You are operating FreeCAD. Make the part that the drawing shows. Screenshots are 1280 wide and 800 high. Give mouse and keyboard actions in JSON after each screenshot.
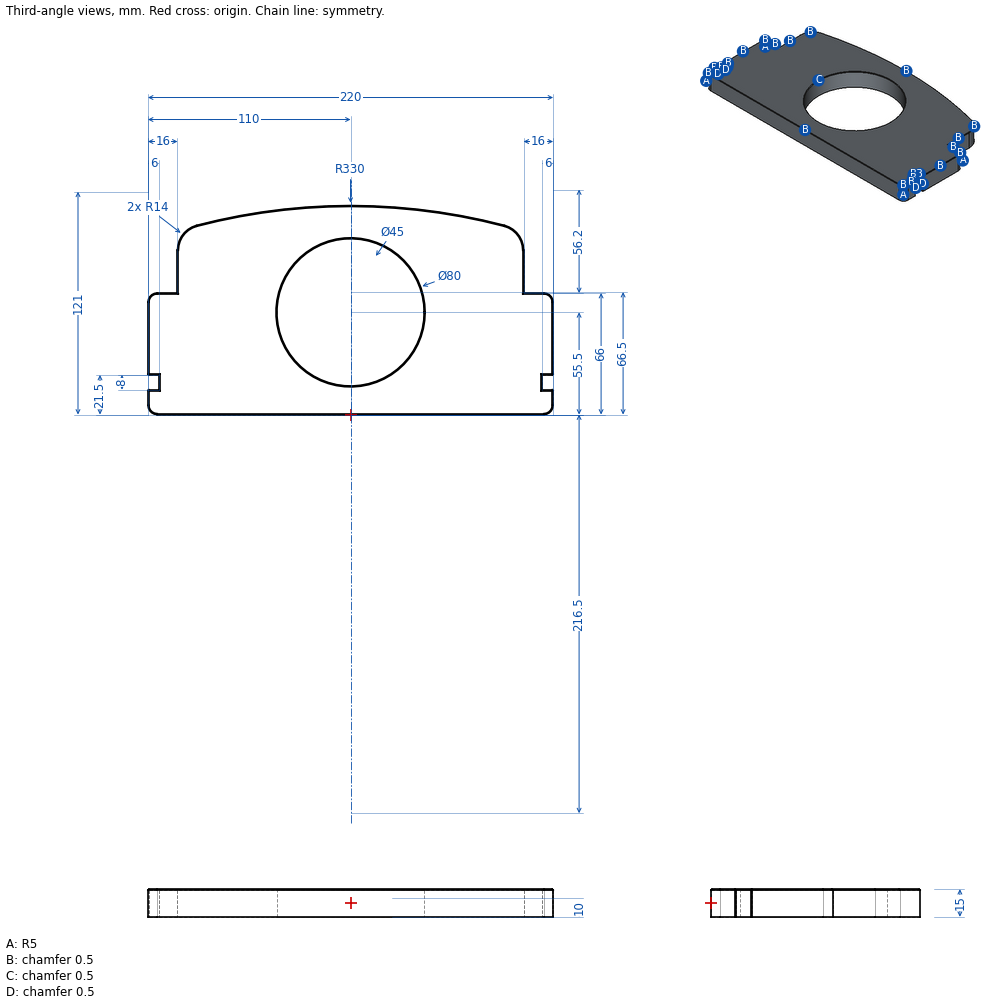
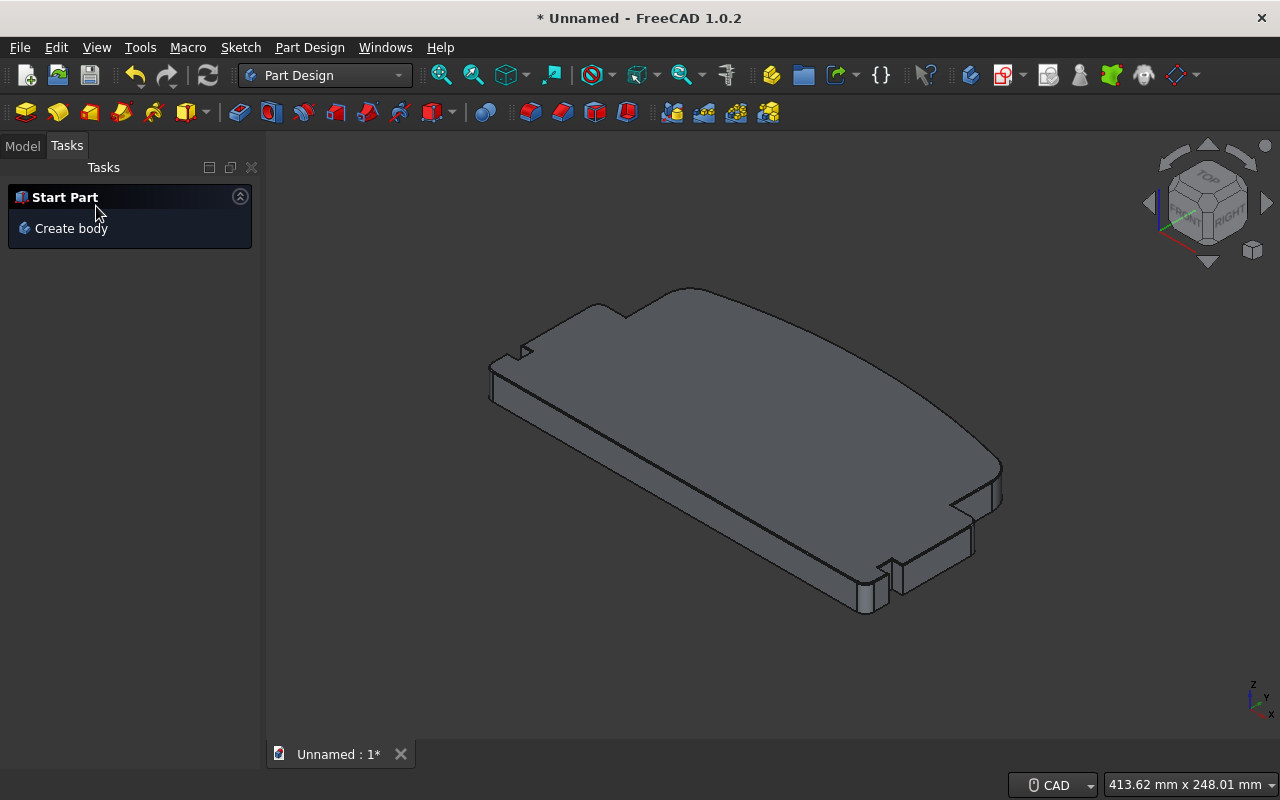
{"action": "left_click", "coordinate": [773, 419]}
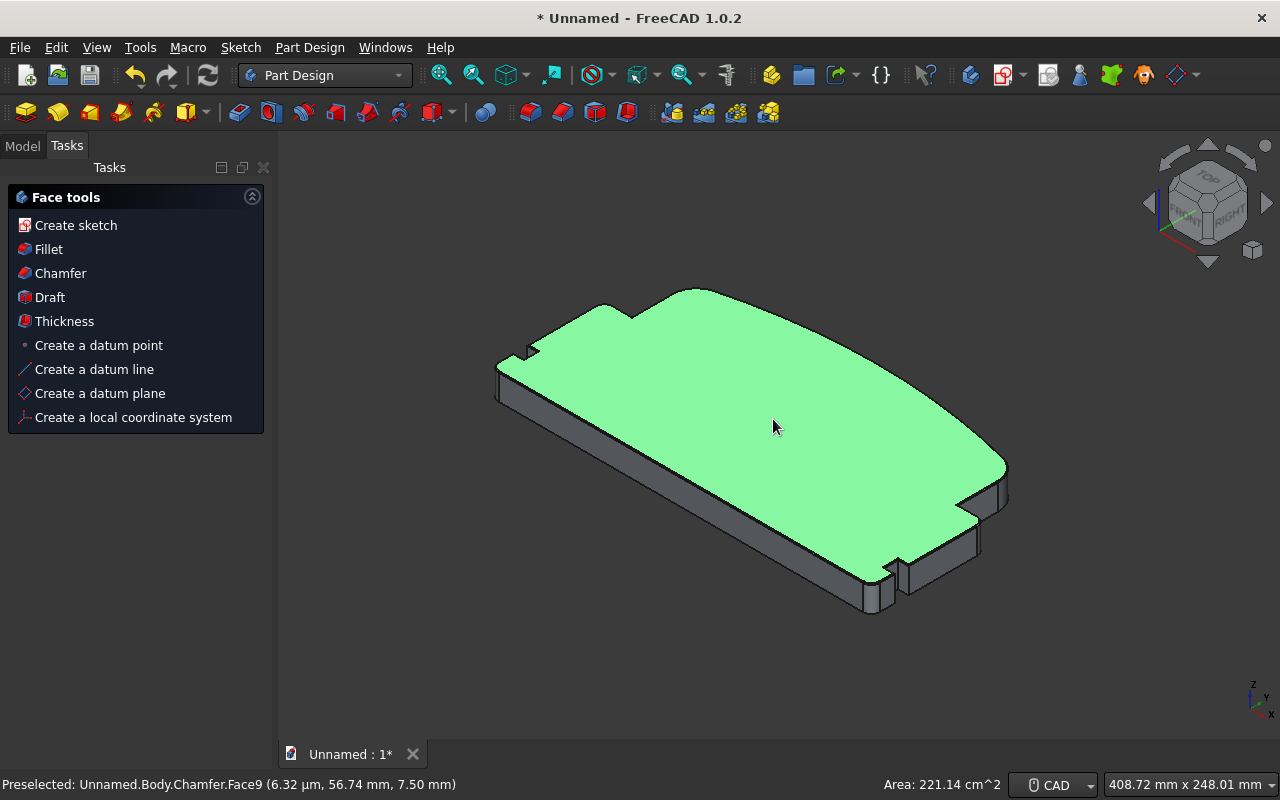
{"action": "left_click", "coordinate": [1004, 76]}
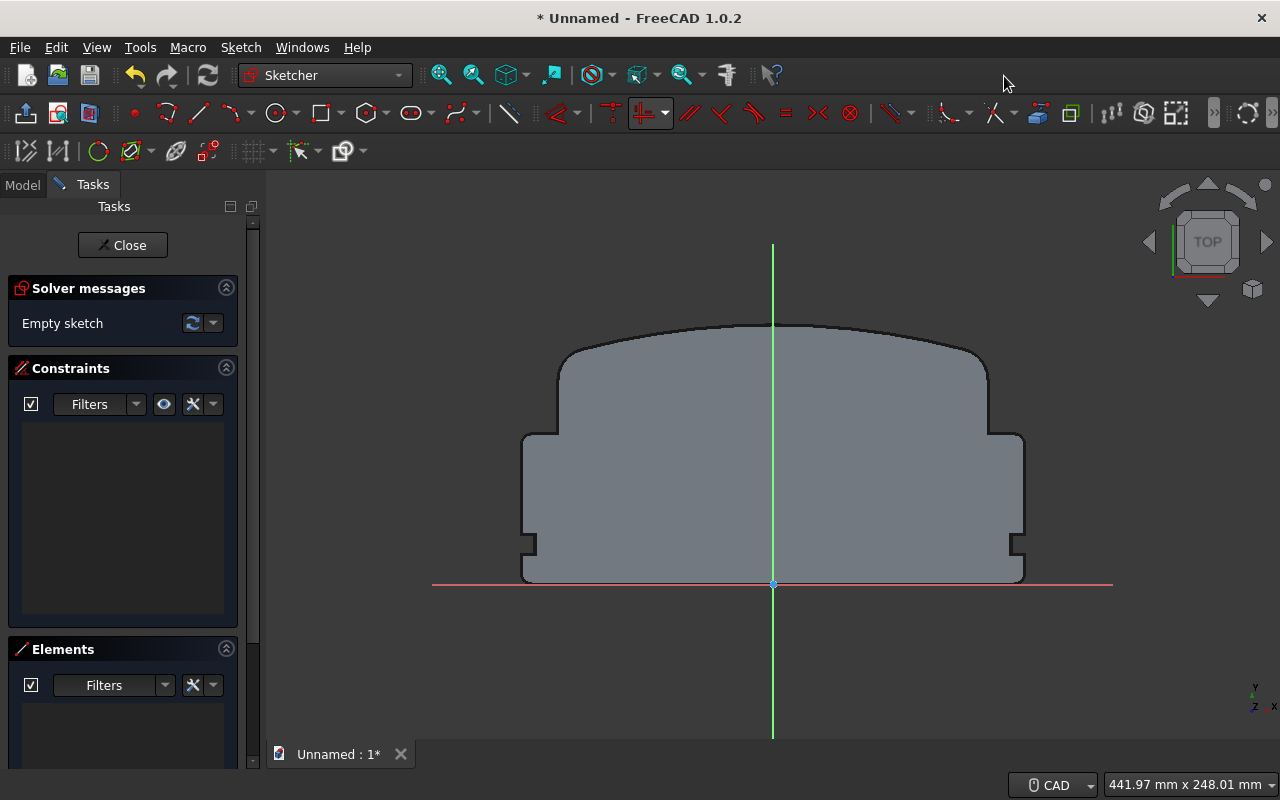
{"action": "scroll", "coordinate": [856, 500], "scroll_direction": "up", "scroll_amount": 3}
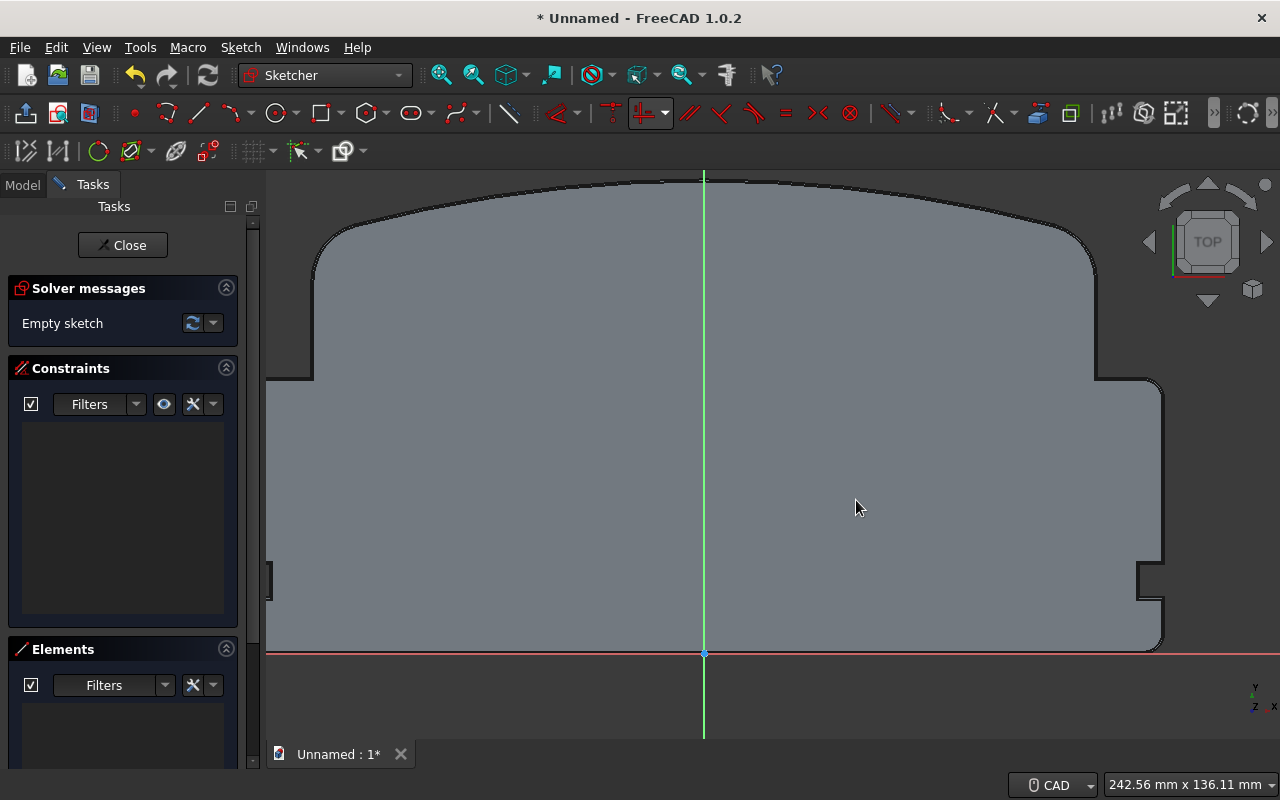
{"action": "left_click", "coordinate": [276, 114]}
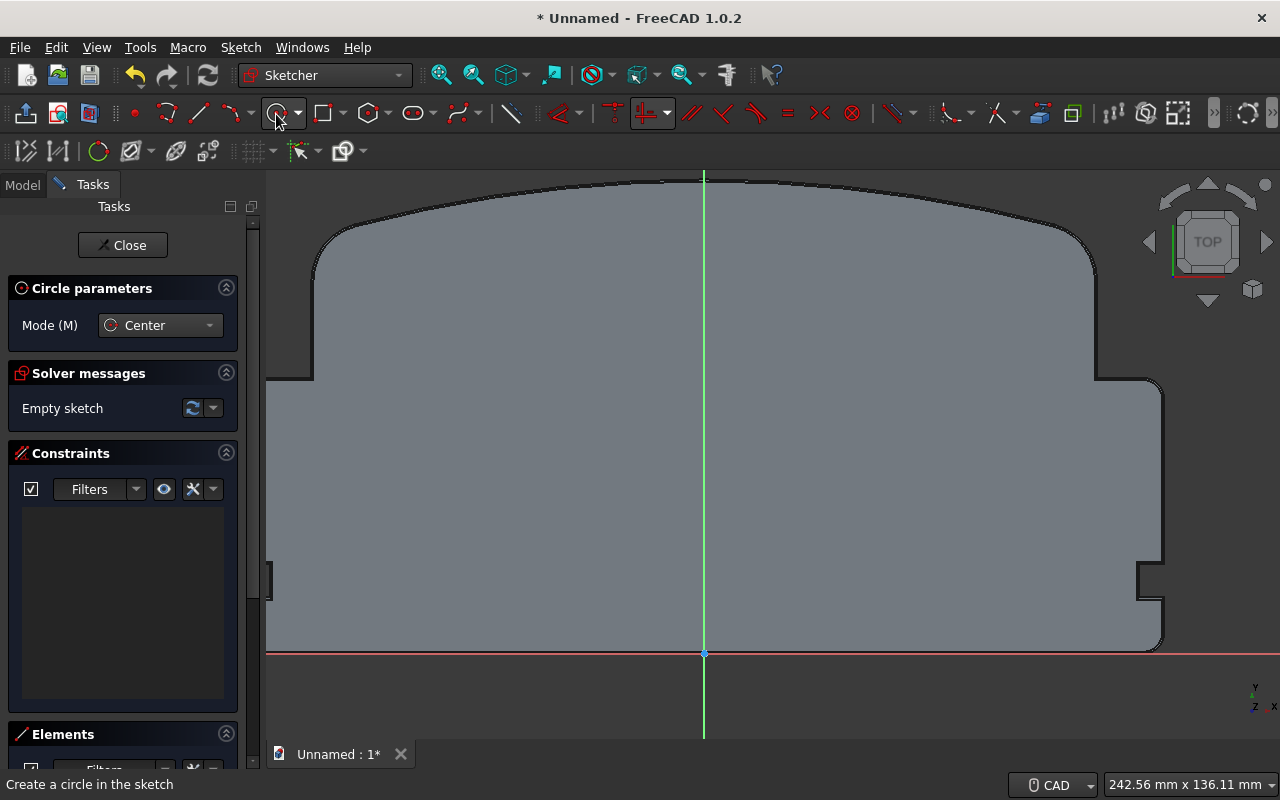
{"action": "left_click", "coordinate": [704, 422]}
{"action": "mouse_move", "coordinate": [823, 304]}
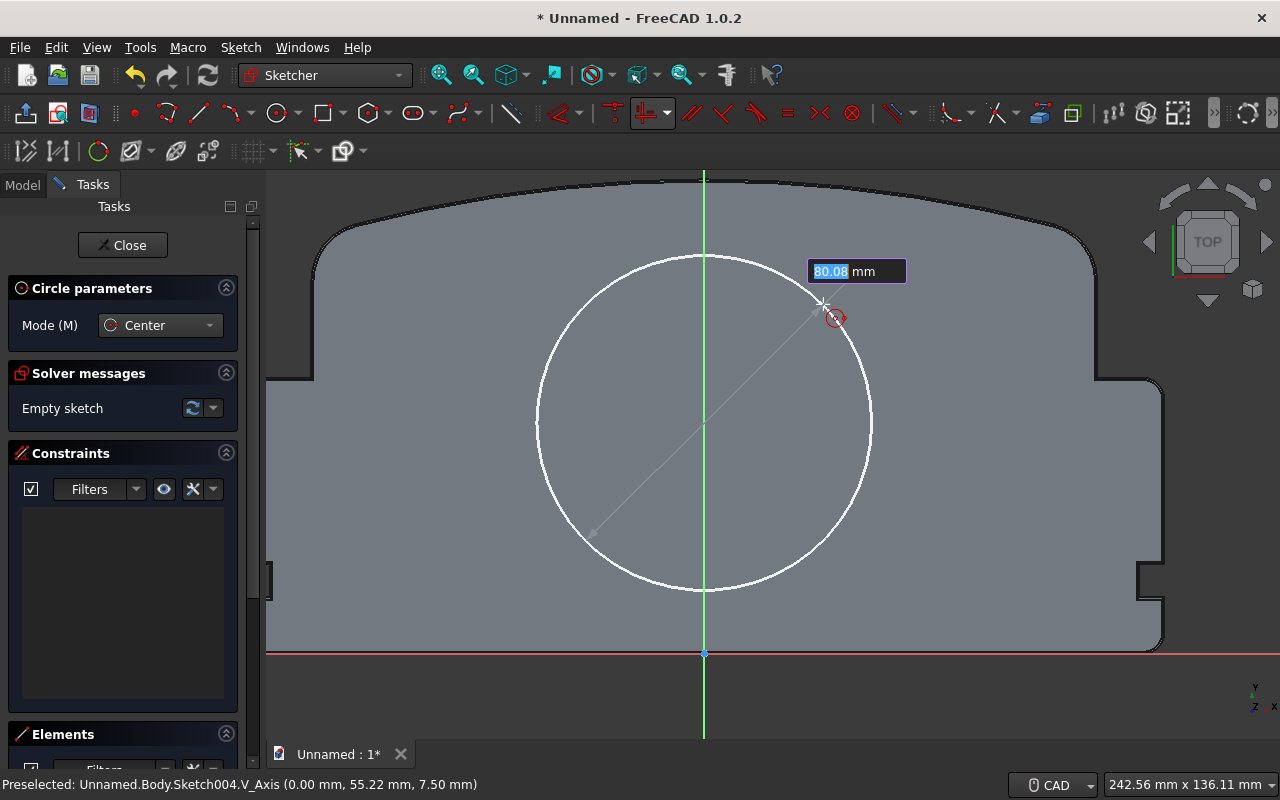
{"action": "type", "text": "80"}
{"action": "key", "text": "Return"}
{"action": "key", "text": "Escape"}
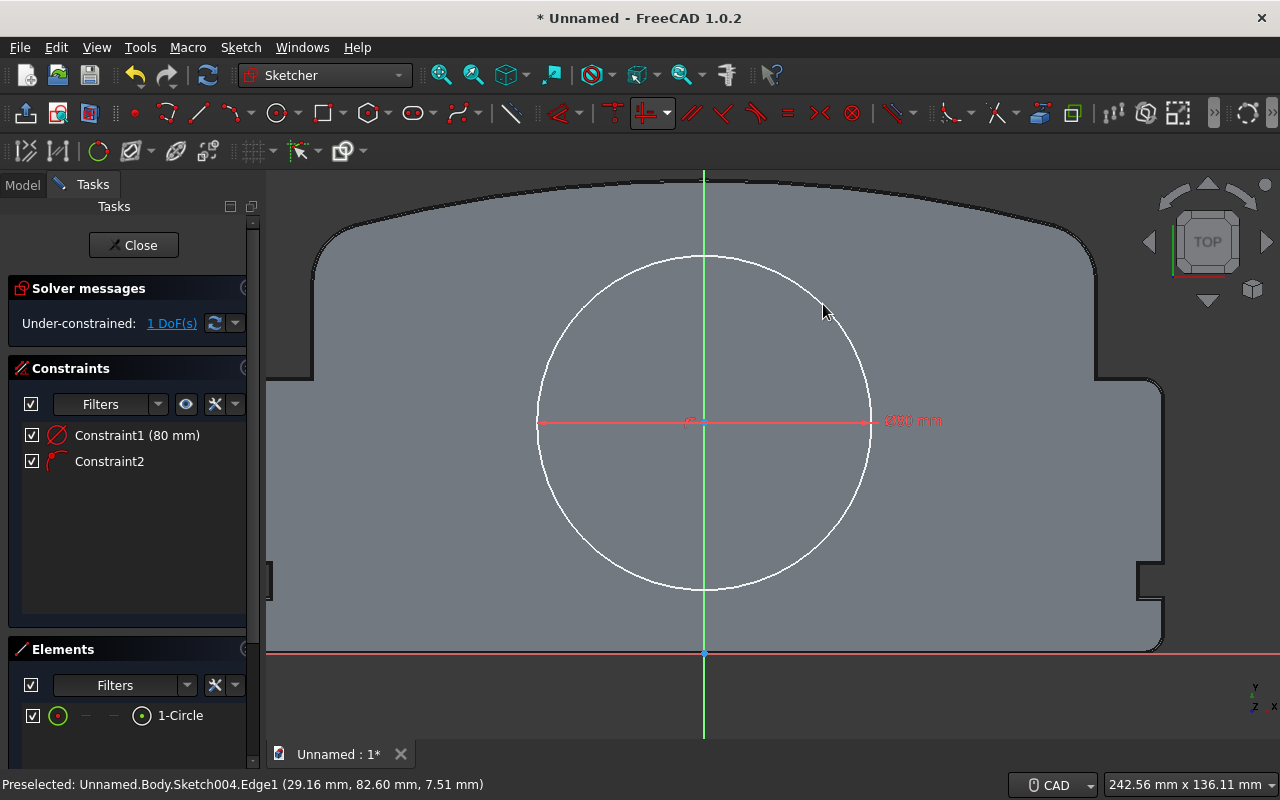
{"action": "left_click", "coordinate": [558, 114]}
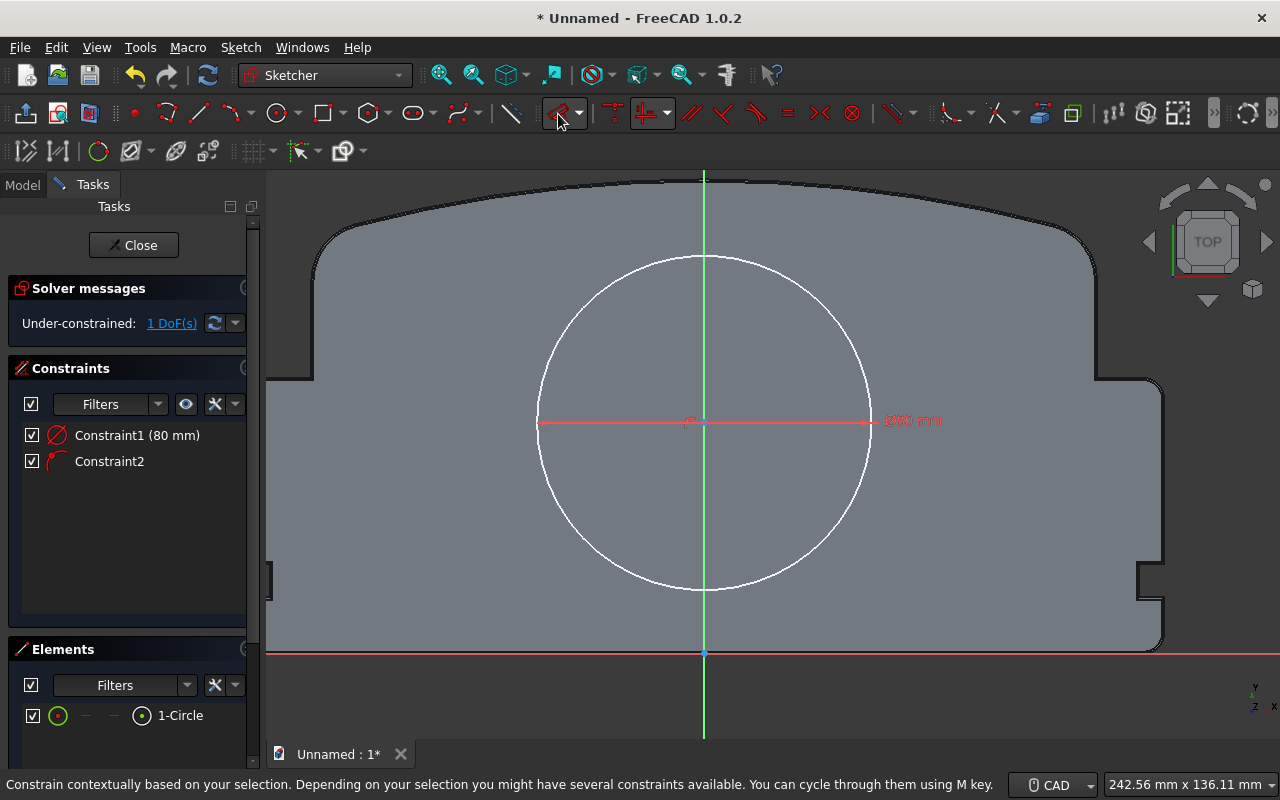
{"action": "left_click", "coordinate": [704, 423]}
{"action": "left_click", "coordinate": [738, 538]}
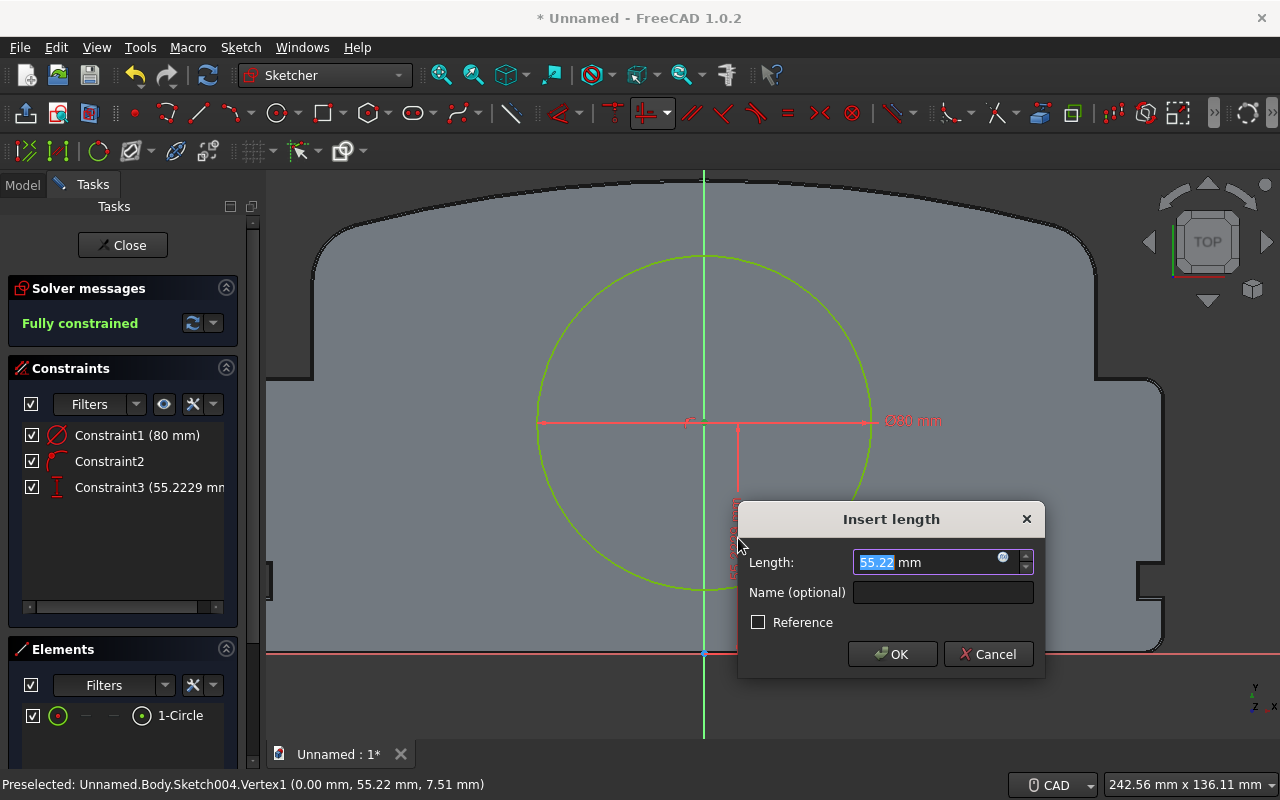
{"action": "type", "text": "55.5"}
{"action": "key", "text": "Return"}
{"action": "key", "text": "Escape"}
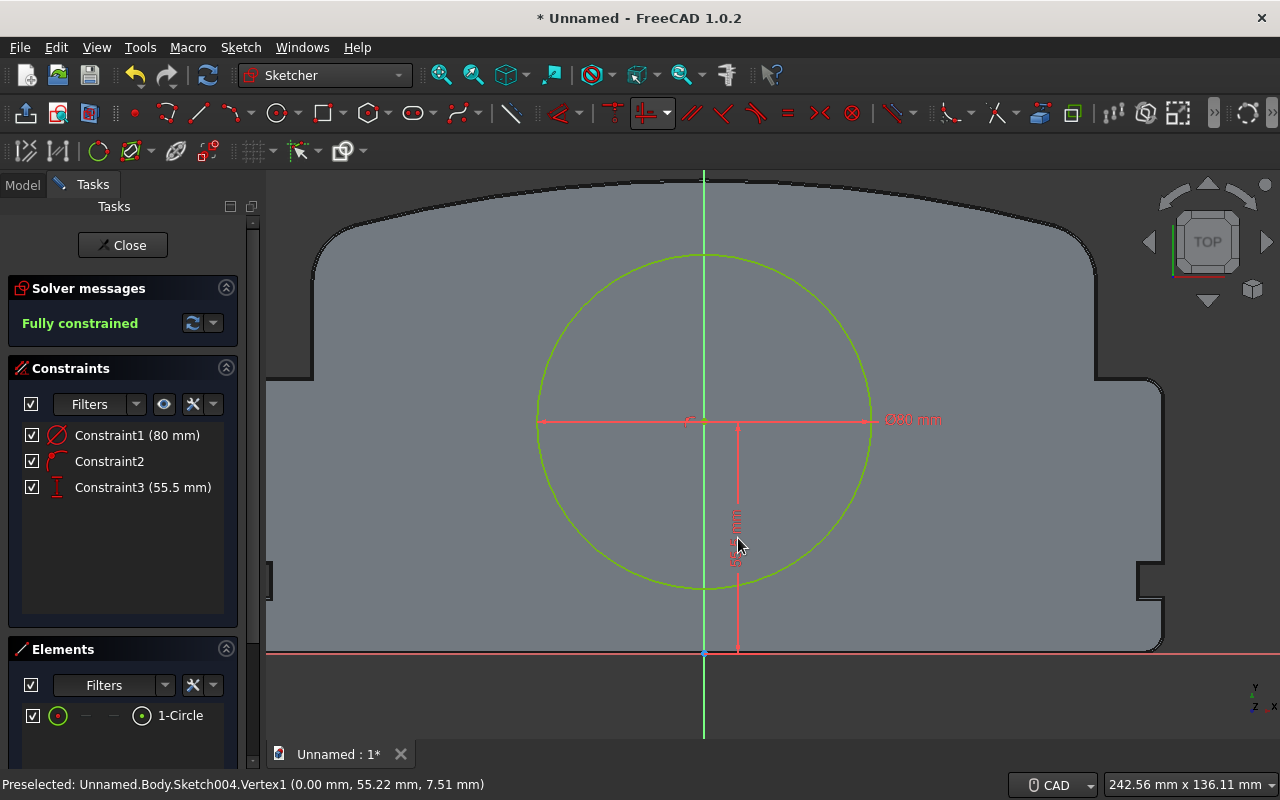
{"action": "left_click", "coordinate": [123, 245]}